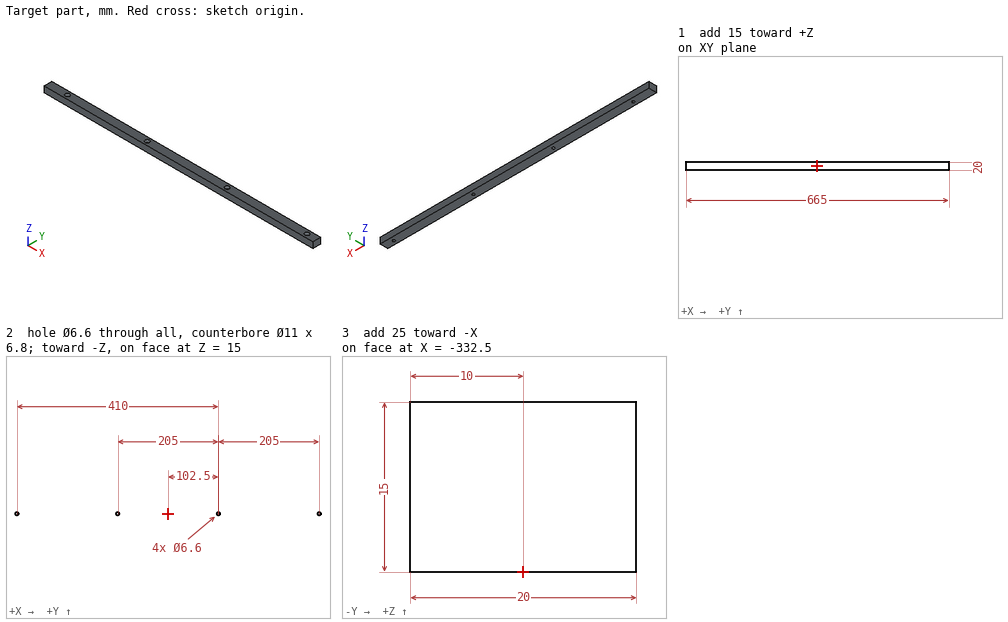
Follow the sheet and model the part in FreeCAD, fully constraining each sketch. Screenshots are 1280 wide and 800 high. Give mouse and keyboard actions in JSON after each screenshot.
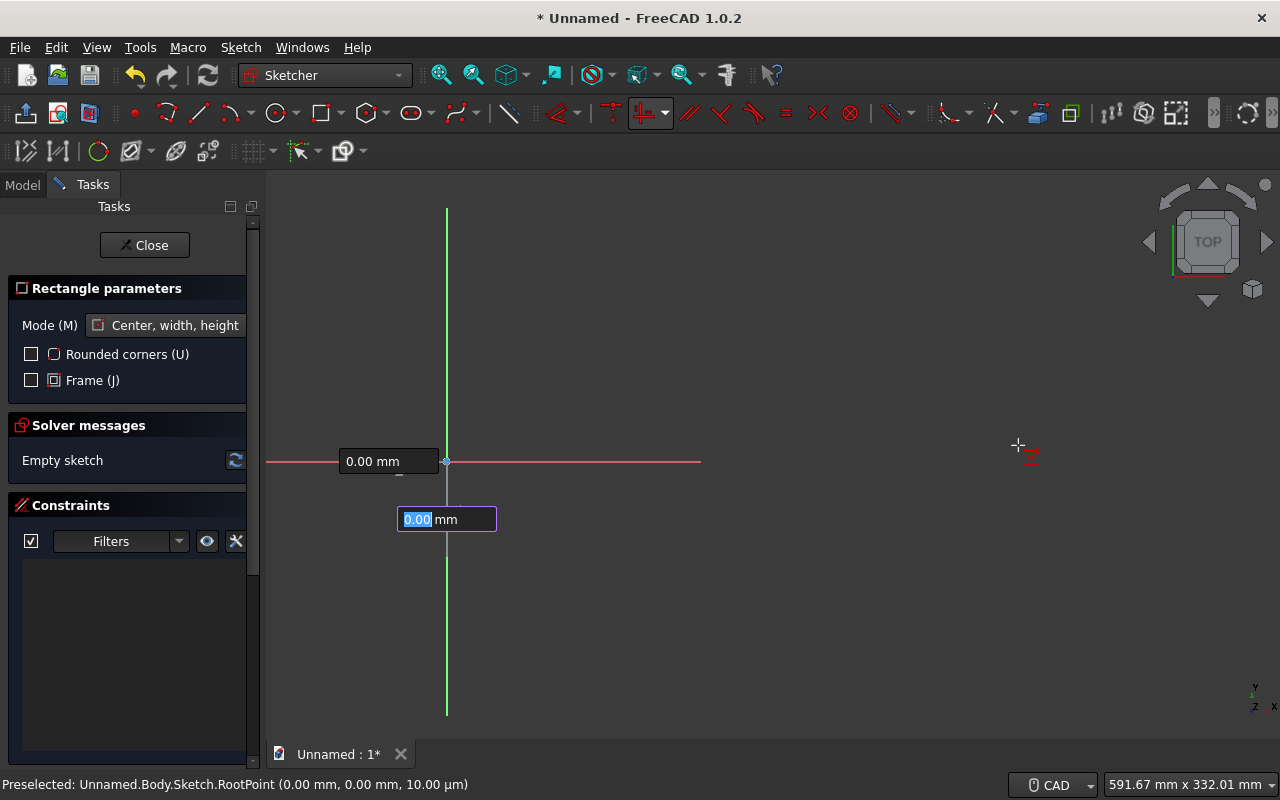
{"action": "left_click", "coordinate": [1017, 445]}
{"action": "key", "text": "Escape"}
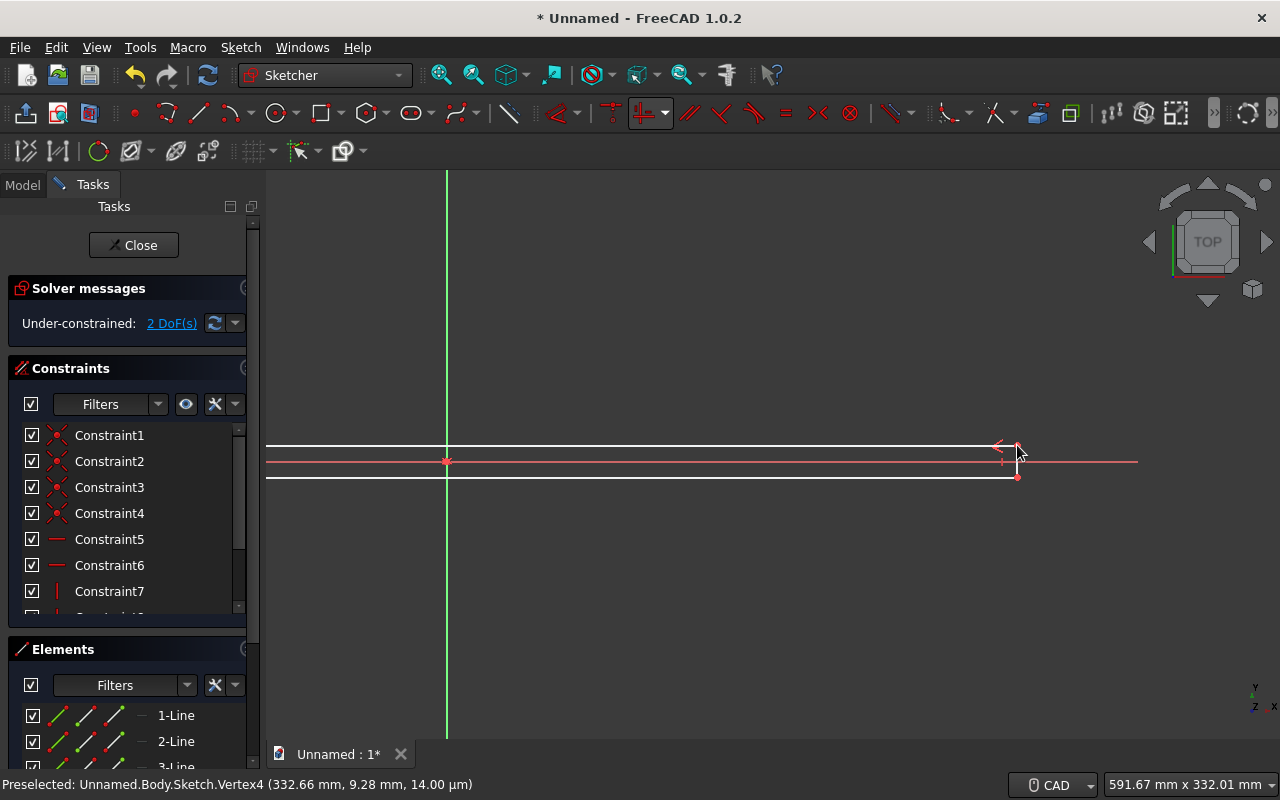
{"action": "left_click", "coordinate": [1017, 465]}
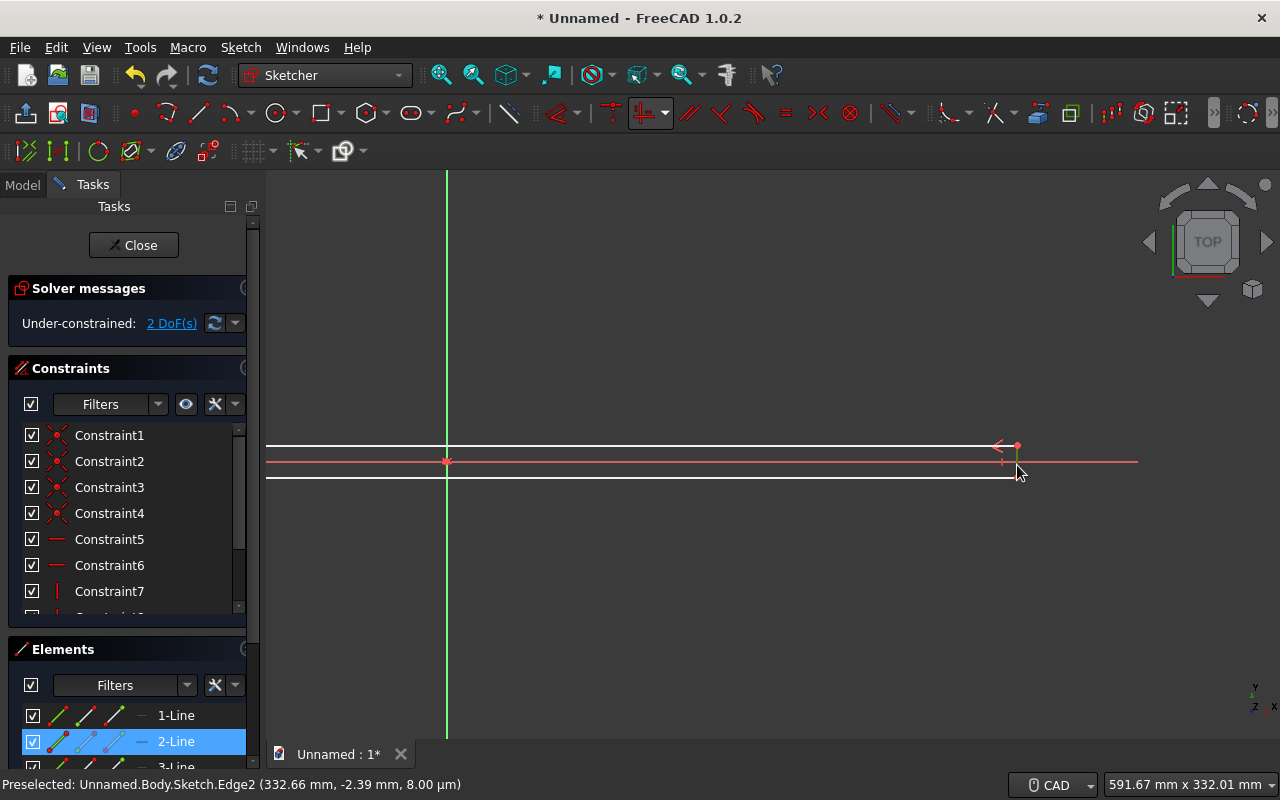
{"action": "key", "text": "i"}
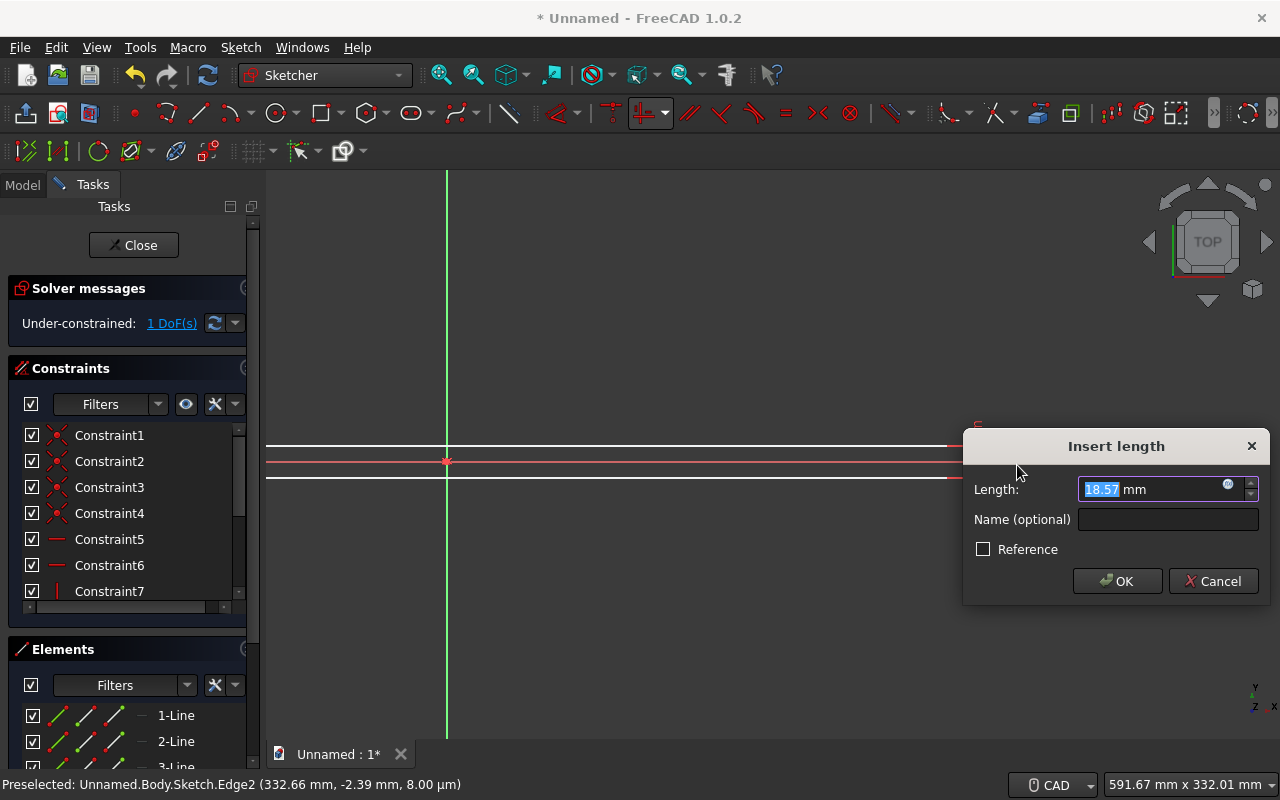
{"action": "type", "text": "20"}
{"action": "key", "text": "Return"}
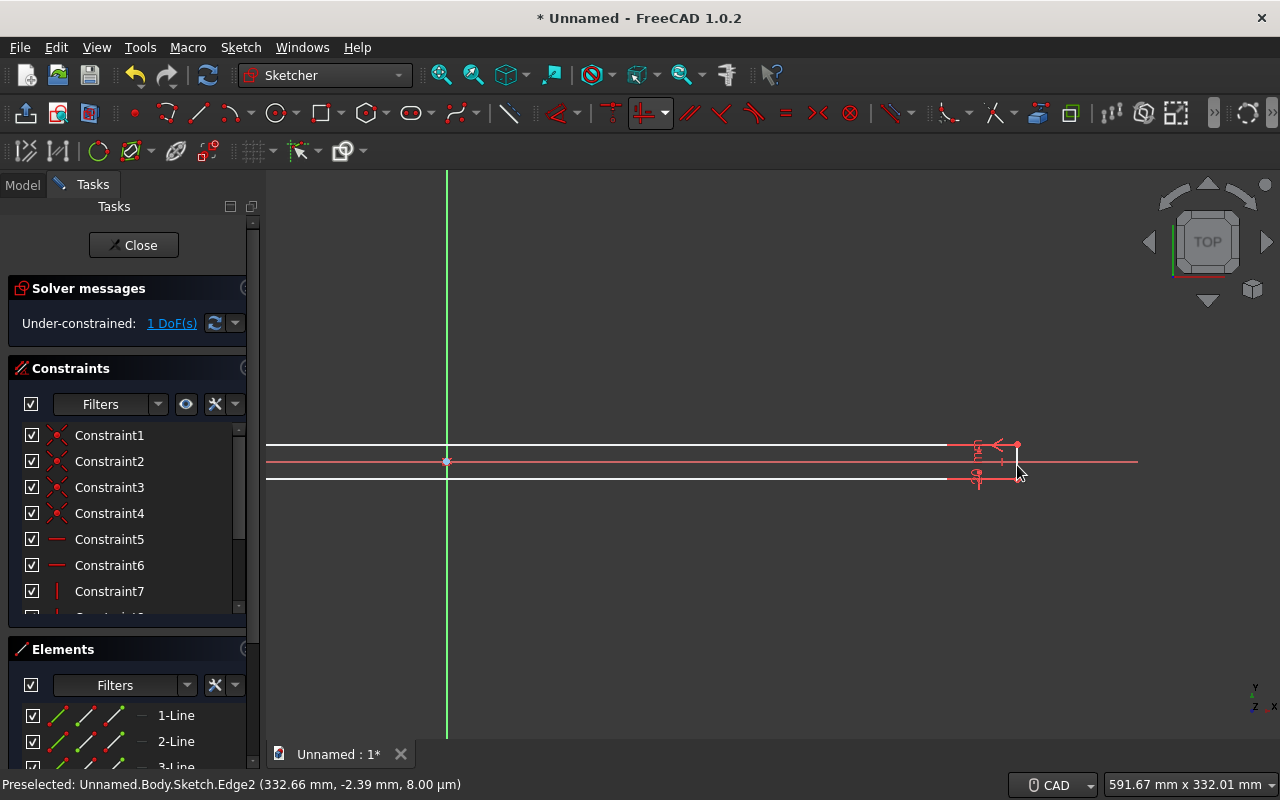
{"action": "left_click", "coordinate": [675, 479]}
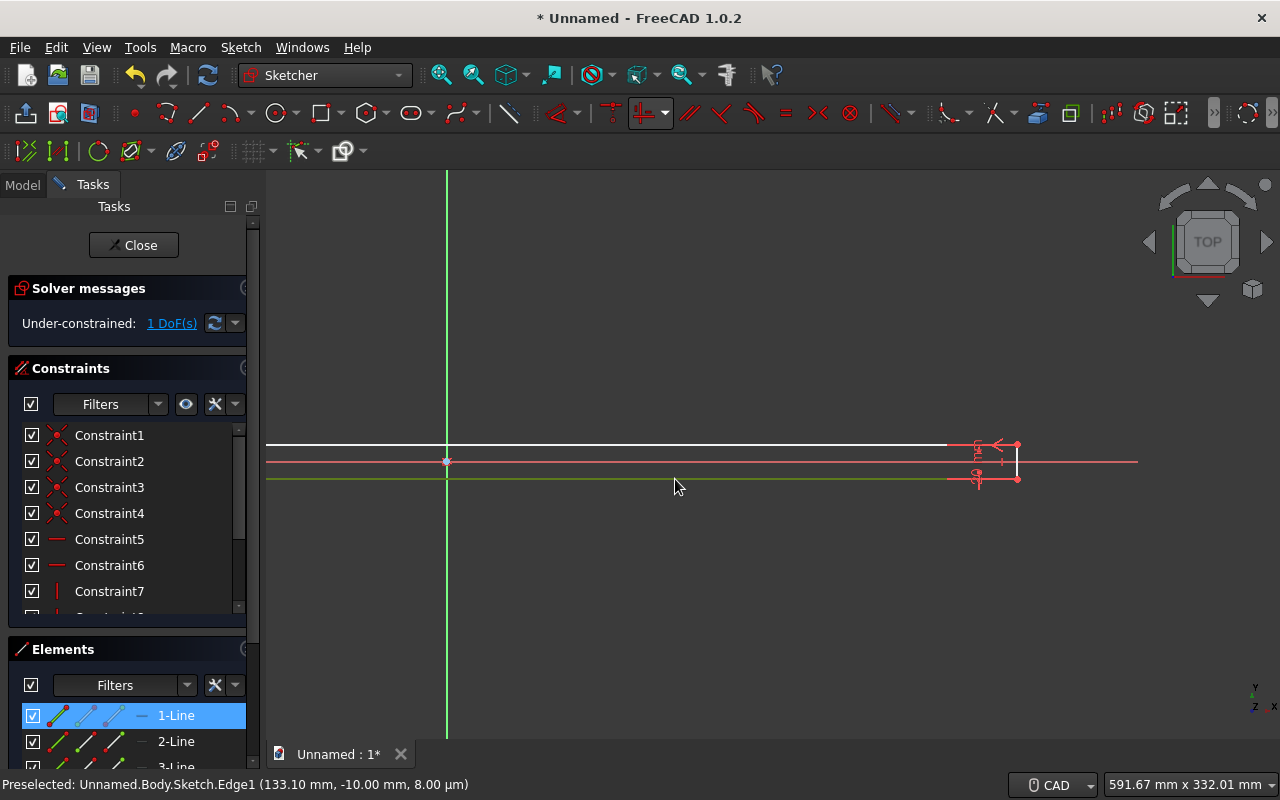
{"action": "key", "text": "l"}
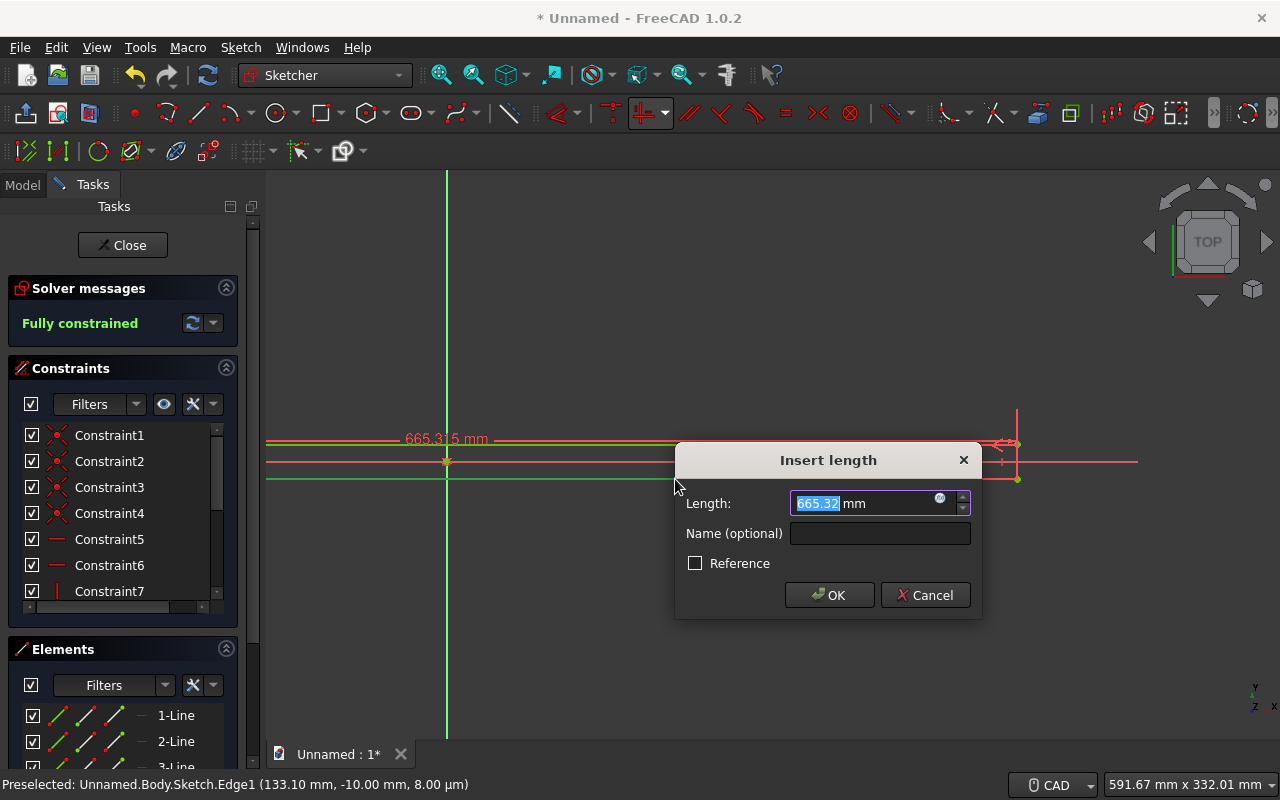
{"action": "type", "text": "665"}
{"action": "key", "text": "Return"}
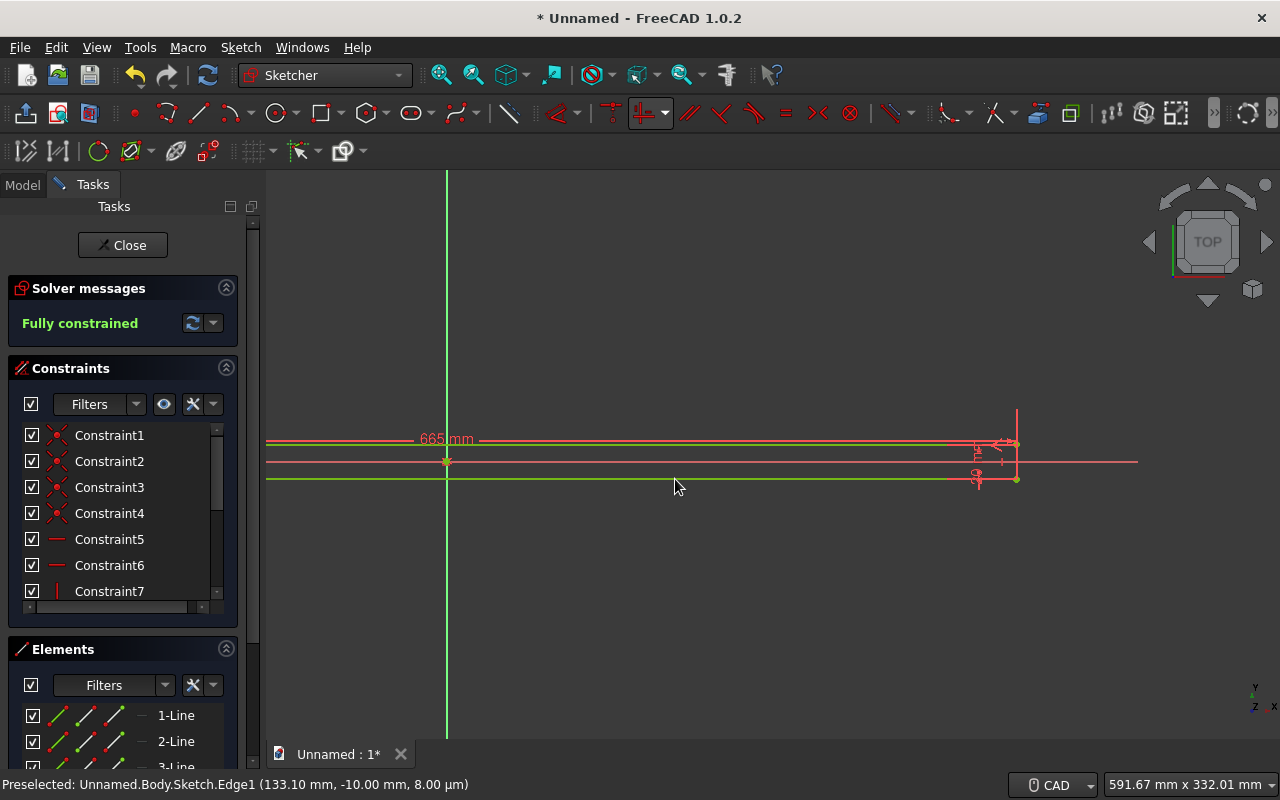
{"action": "left_click", "coordinate": [123, 245]}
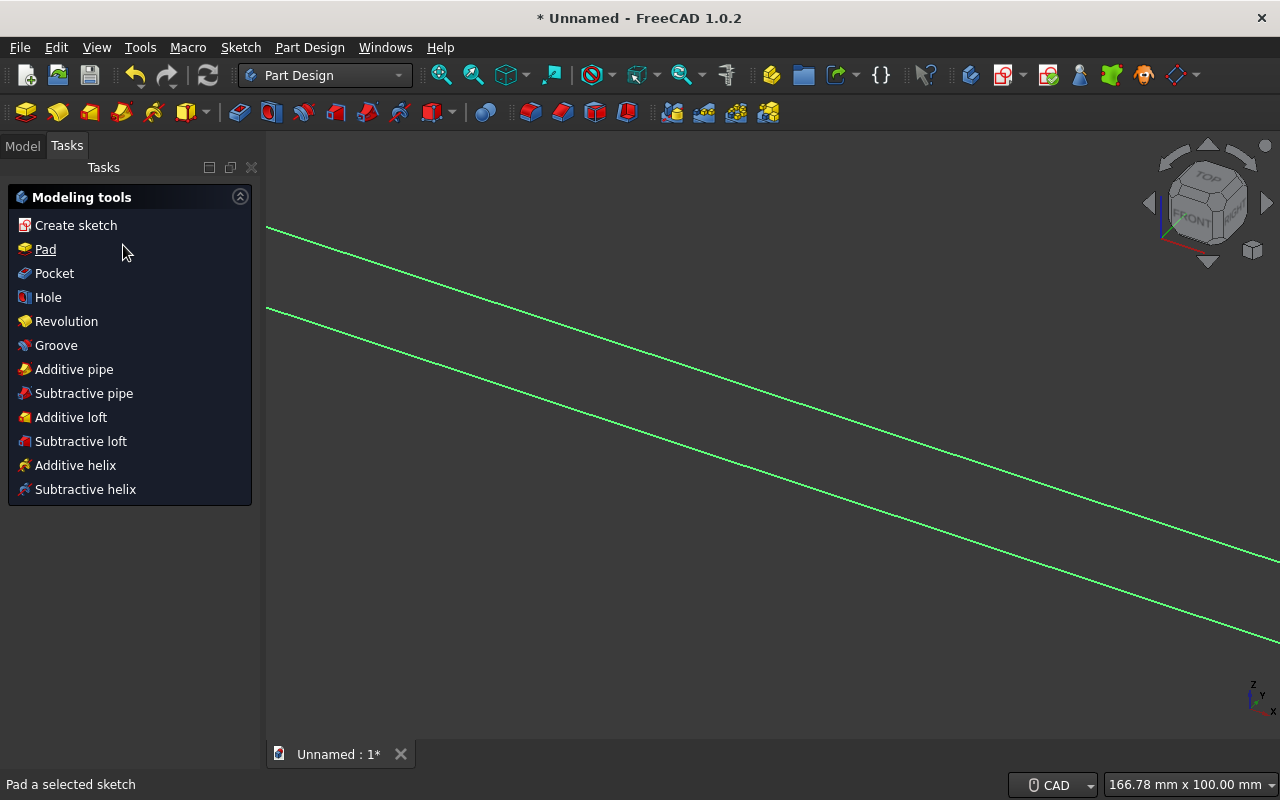
{"action": "left_click", "coordinate": [26, 112]}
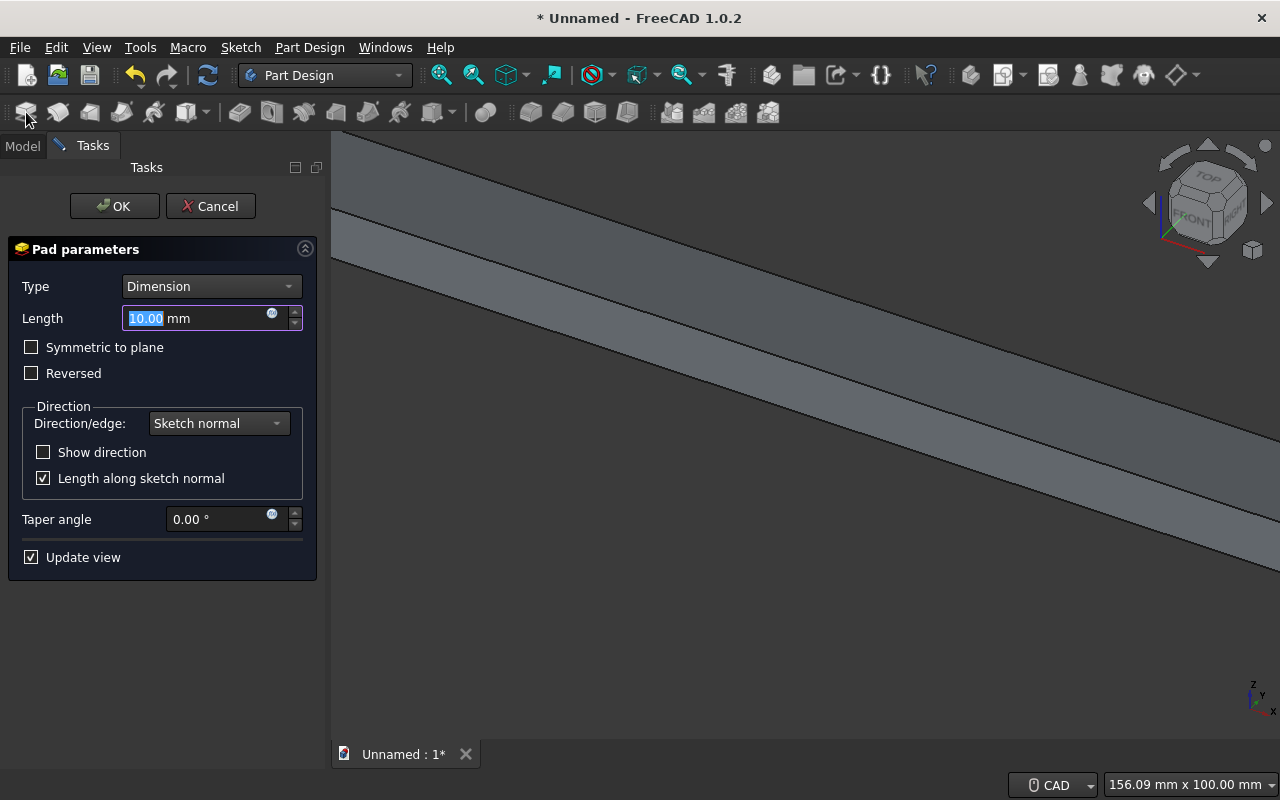
{"action": "type", "text": "15"}
{"action": "key", "text": "Tab"}